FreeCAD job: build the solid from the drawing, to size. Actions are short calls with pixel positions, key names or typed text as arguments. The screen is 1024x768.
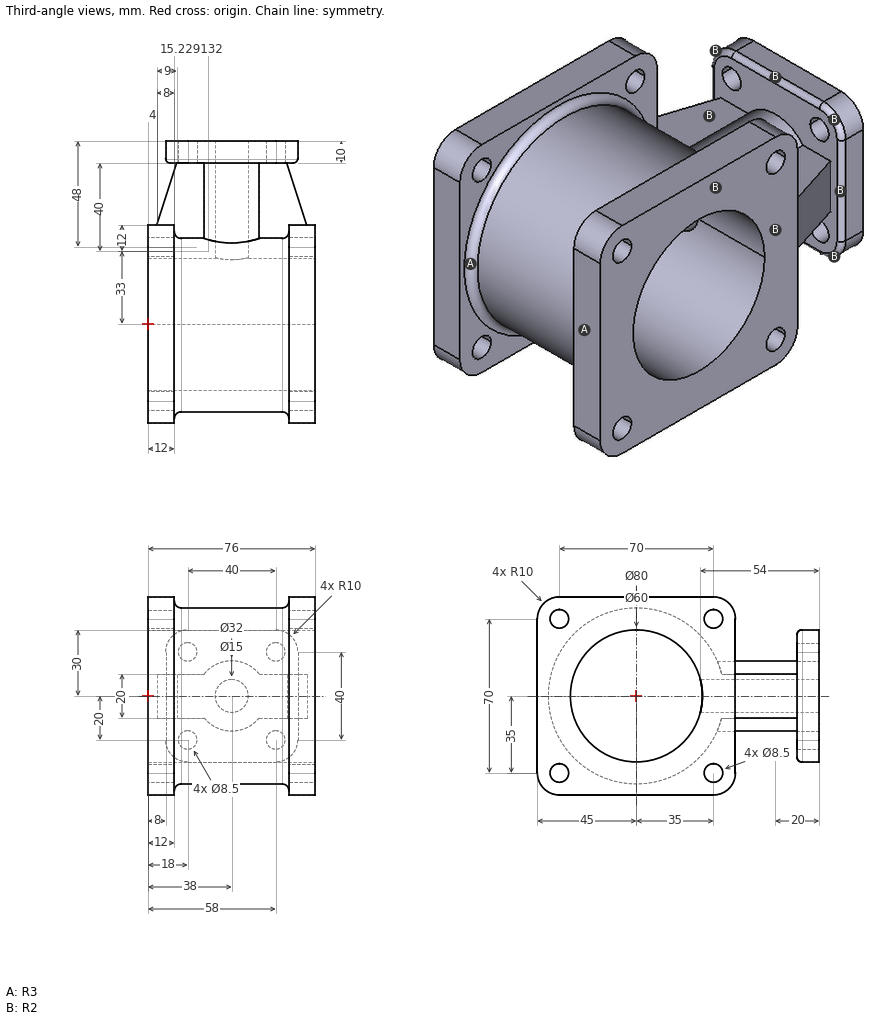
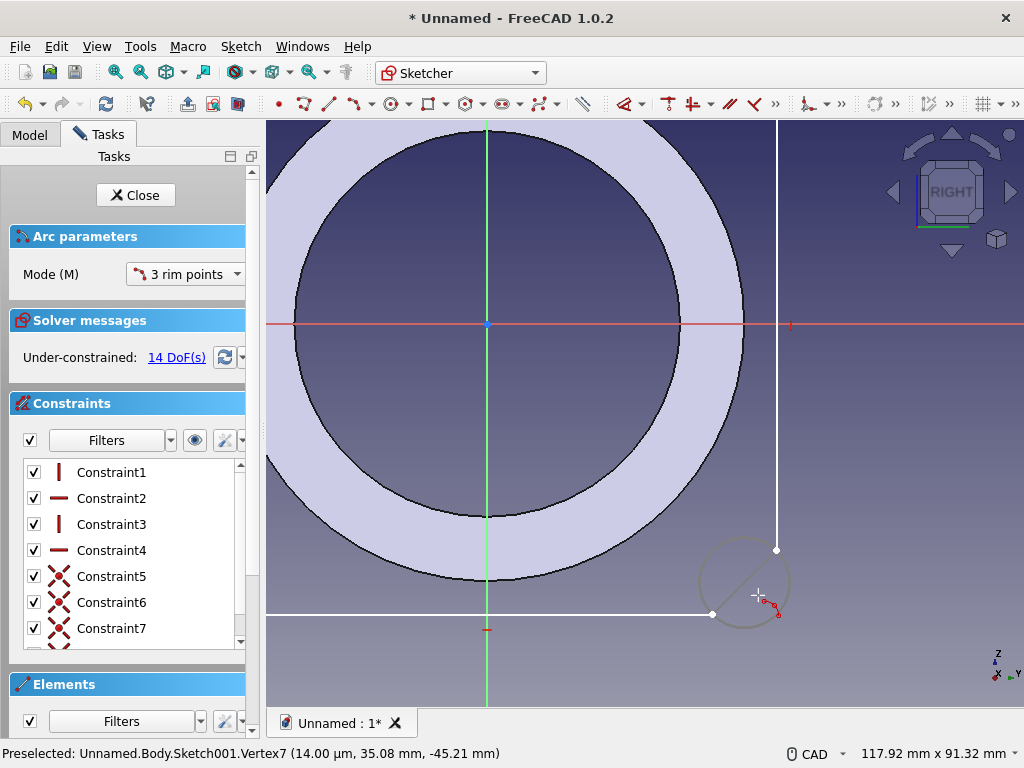
click(758, 594)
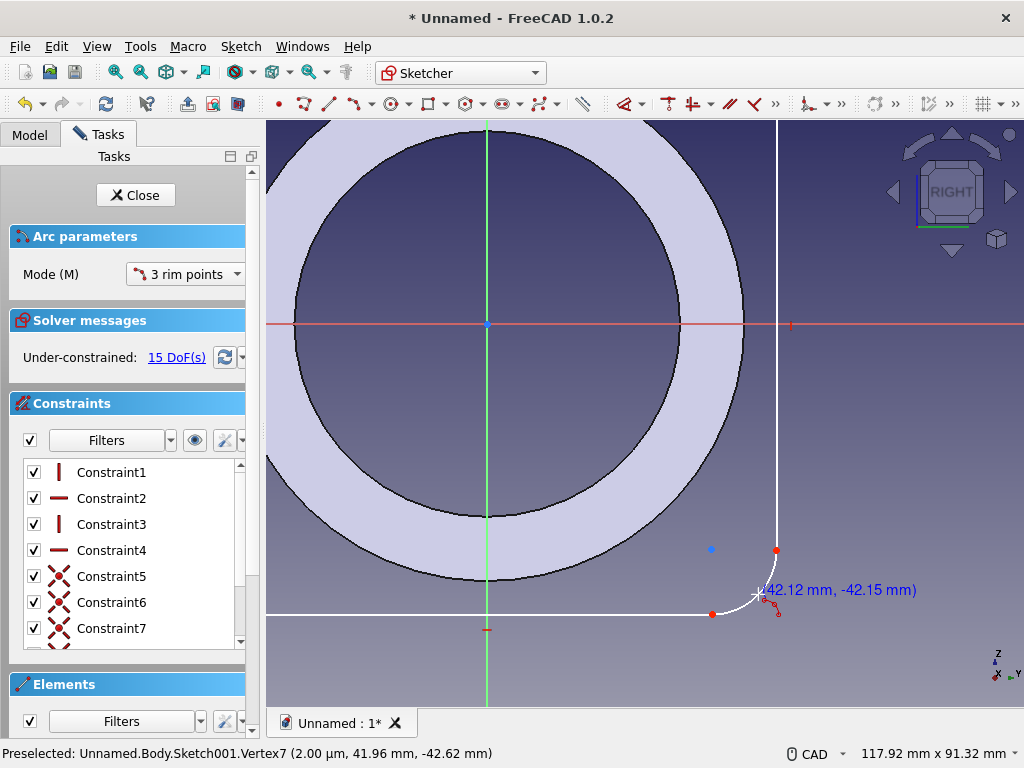
scroll(758, 595, down, 2)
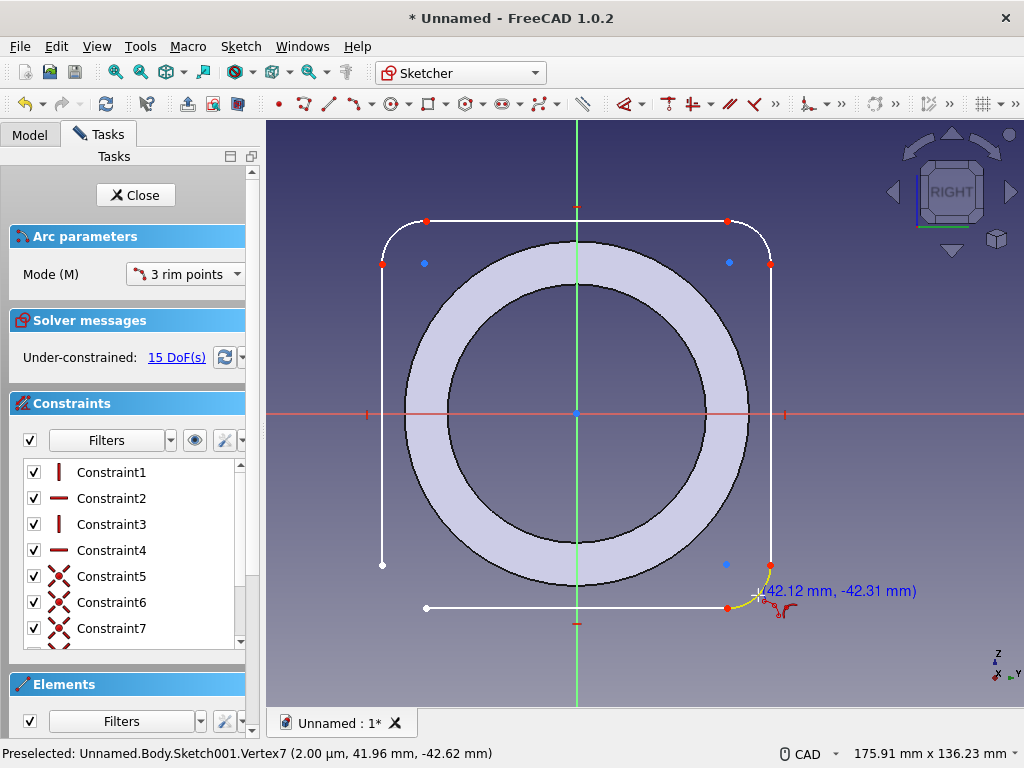
click(426, 608)
click(382, 566)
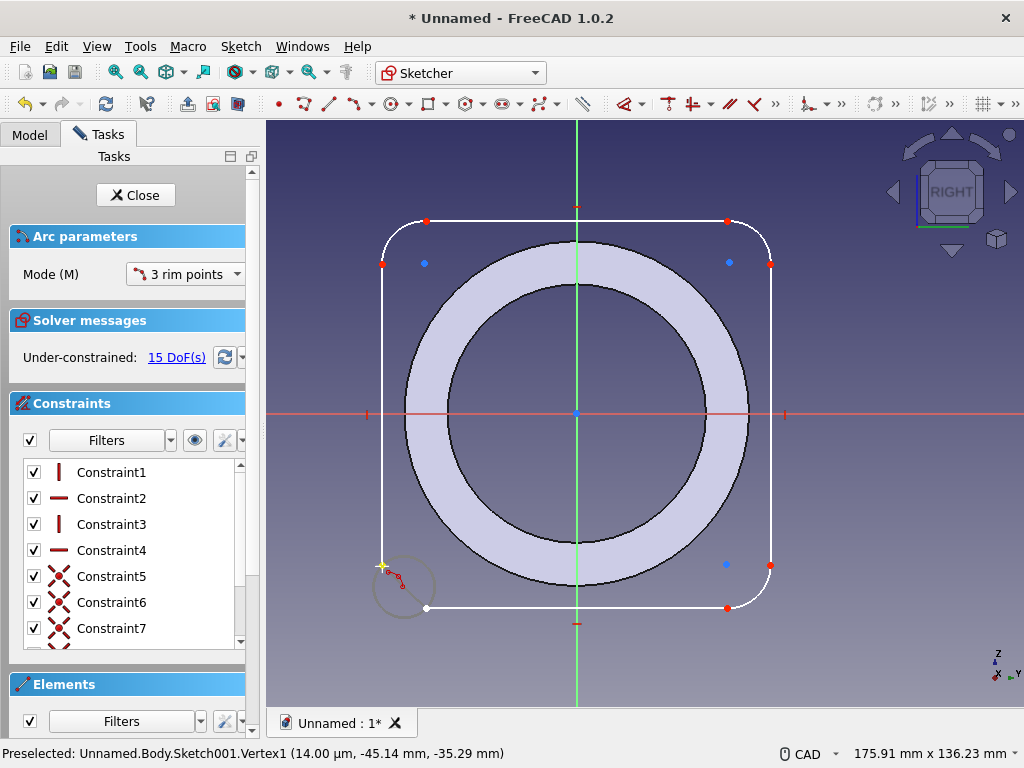
scroll(395, 595, up, 2)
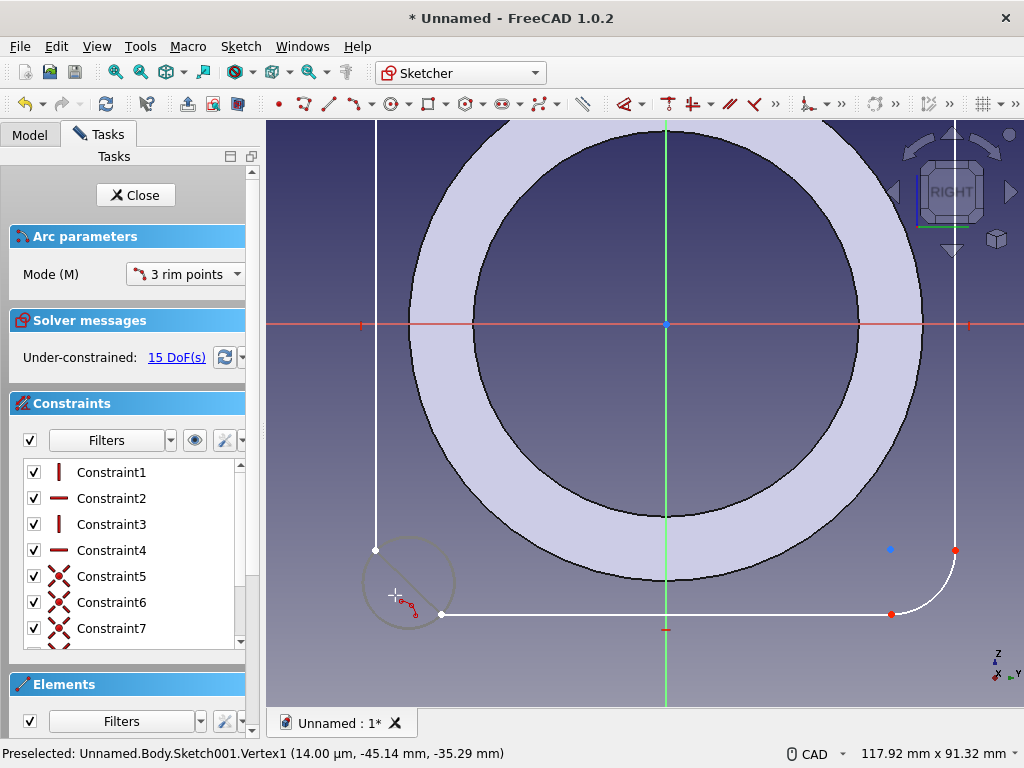
click(396, 594)
key(Escape)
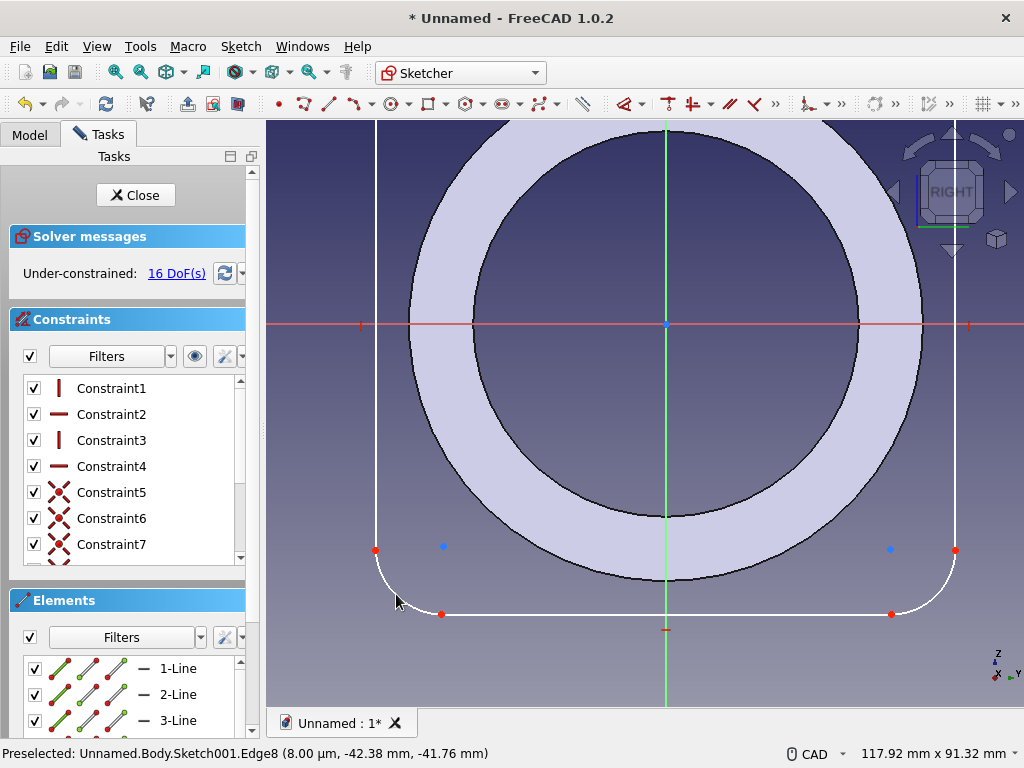
click(376, 416)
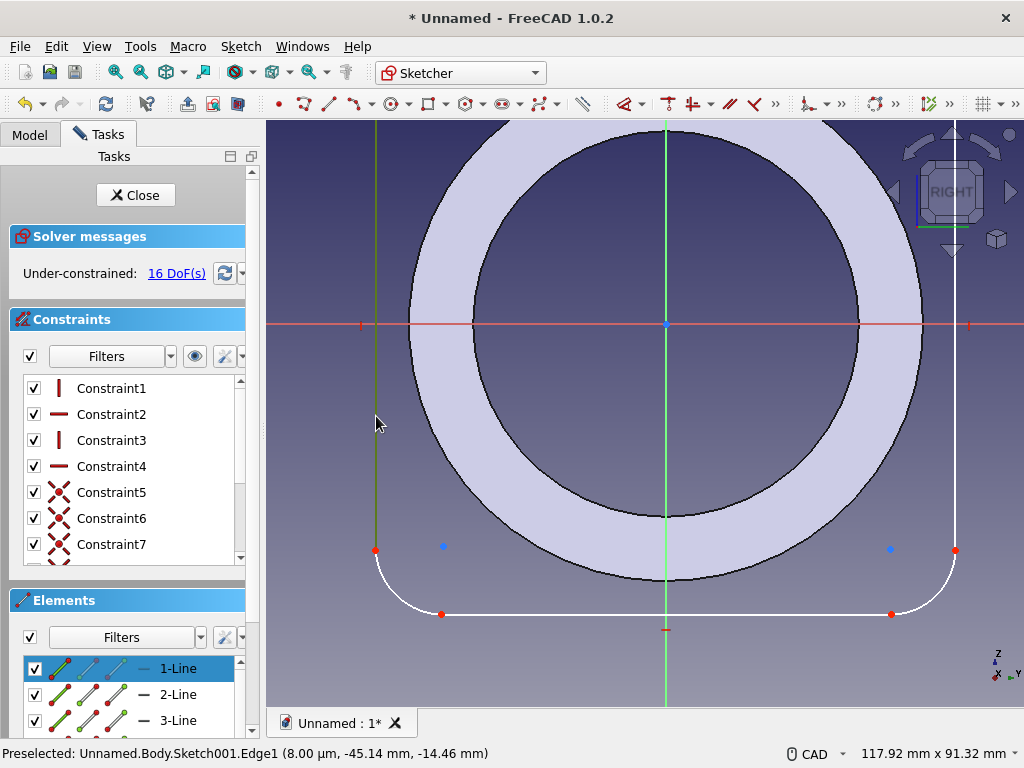
scroll(395, 595, down, 2)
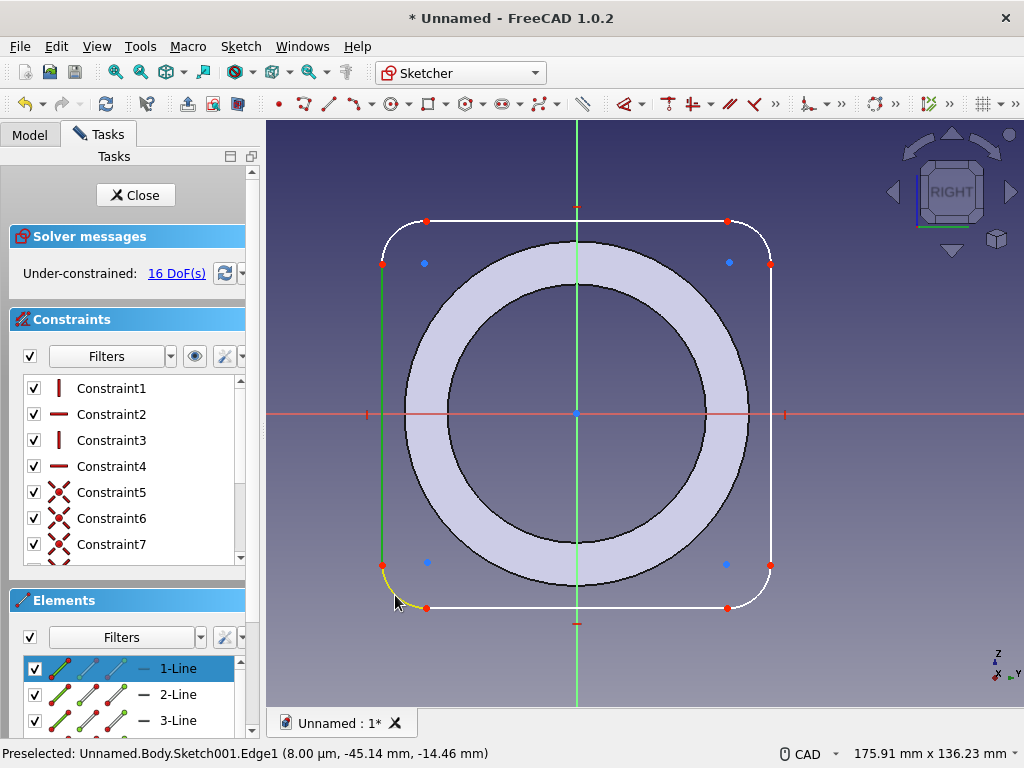
click(406, 225)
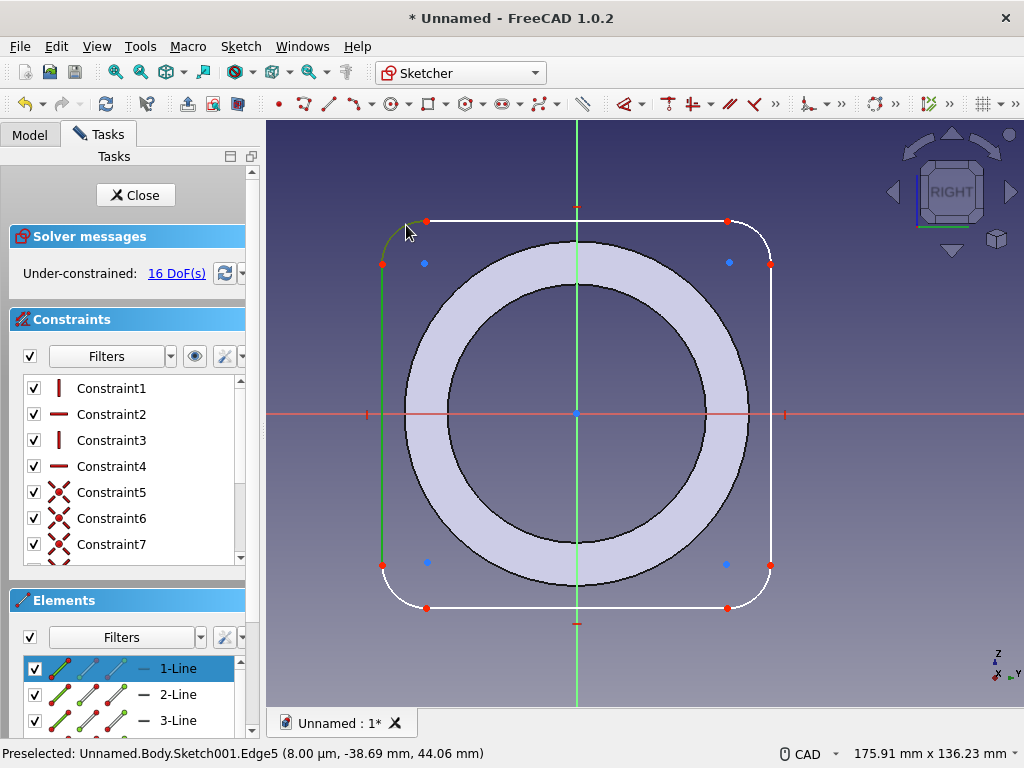
key(t)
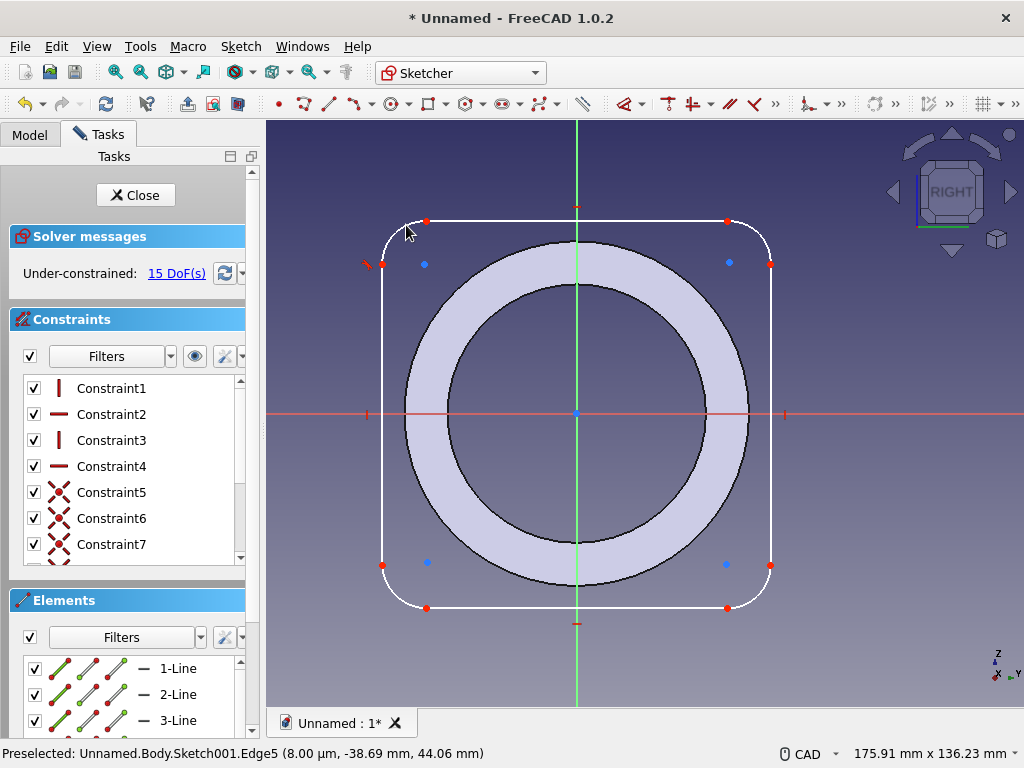
click(382, 475)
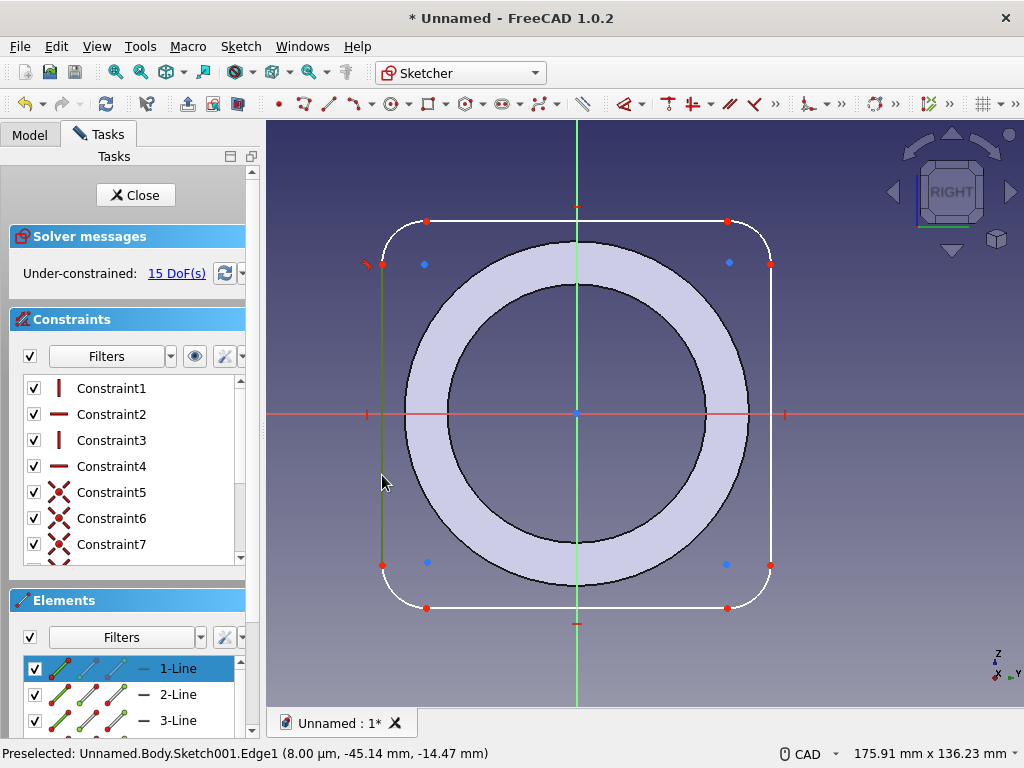
click(388, 585)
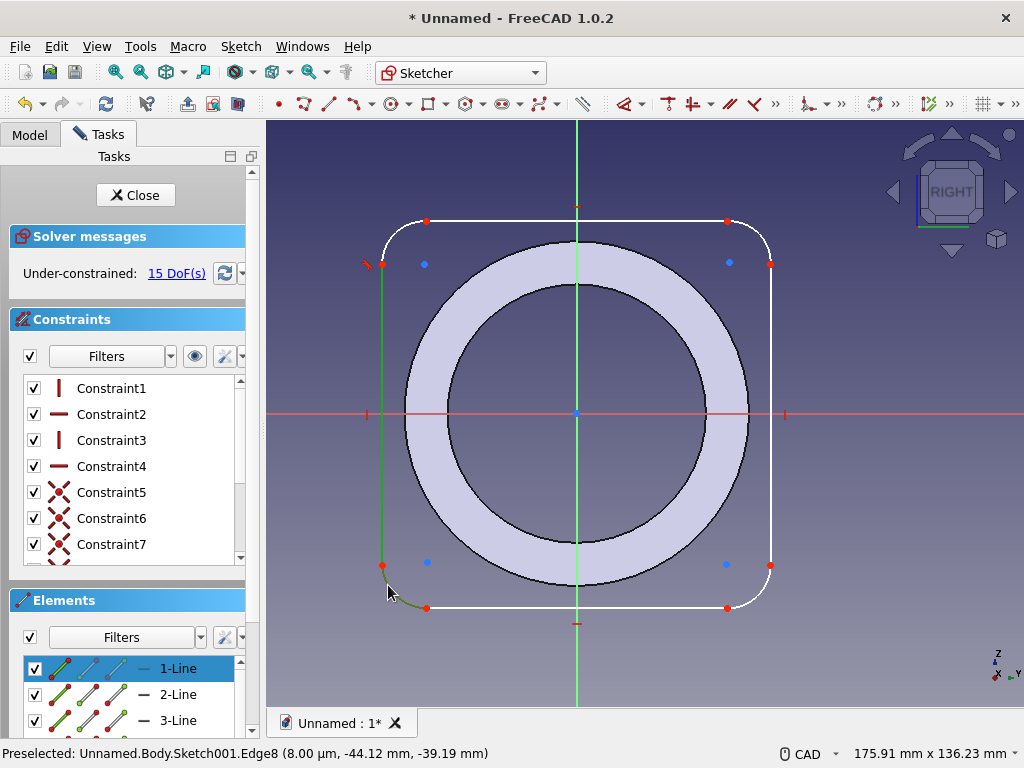
key(t)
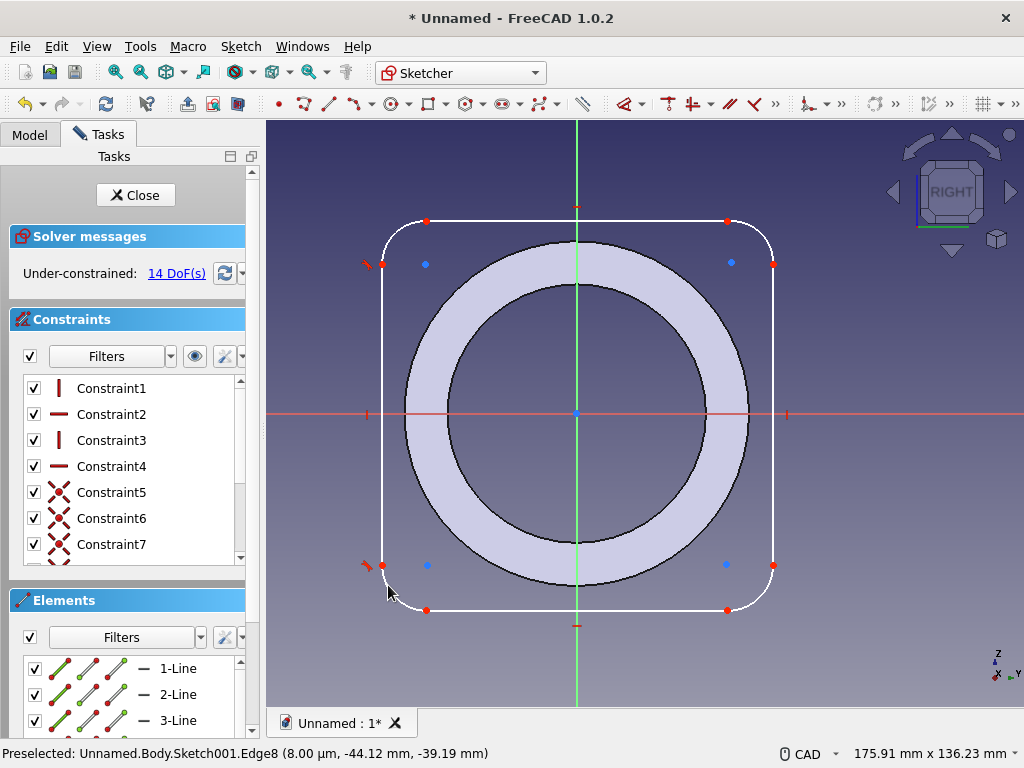
click(517, 221)